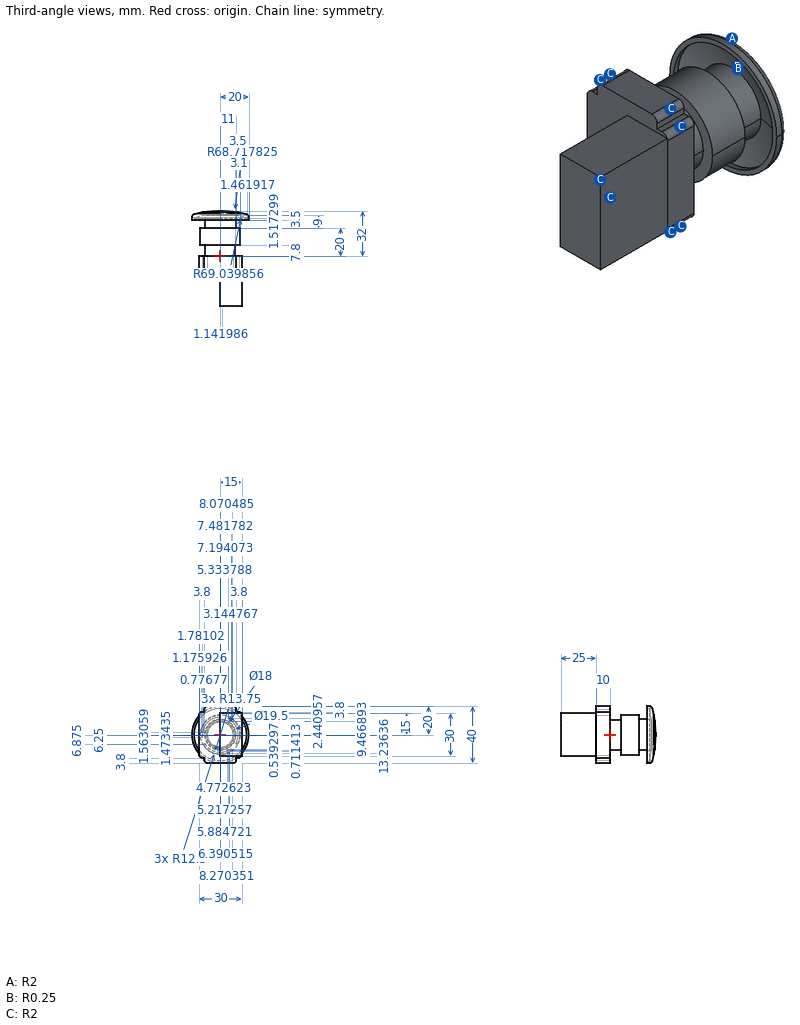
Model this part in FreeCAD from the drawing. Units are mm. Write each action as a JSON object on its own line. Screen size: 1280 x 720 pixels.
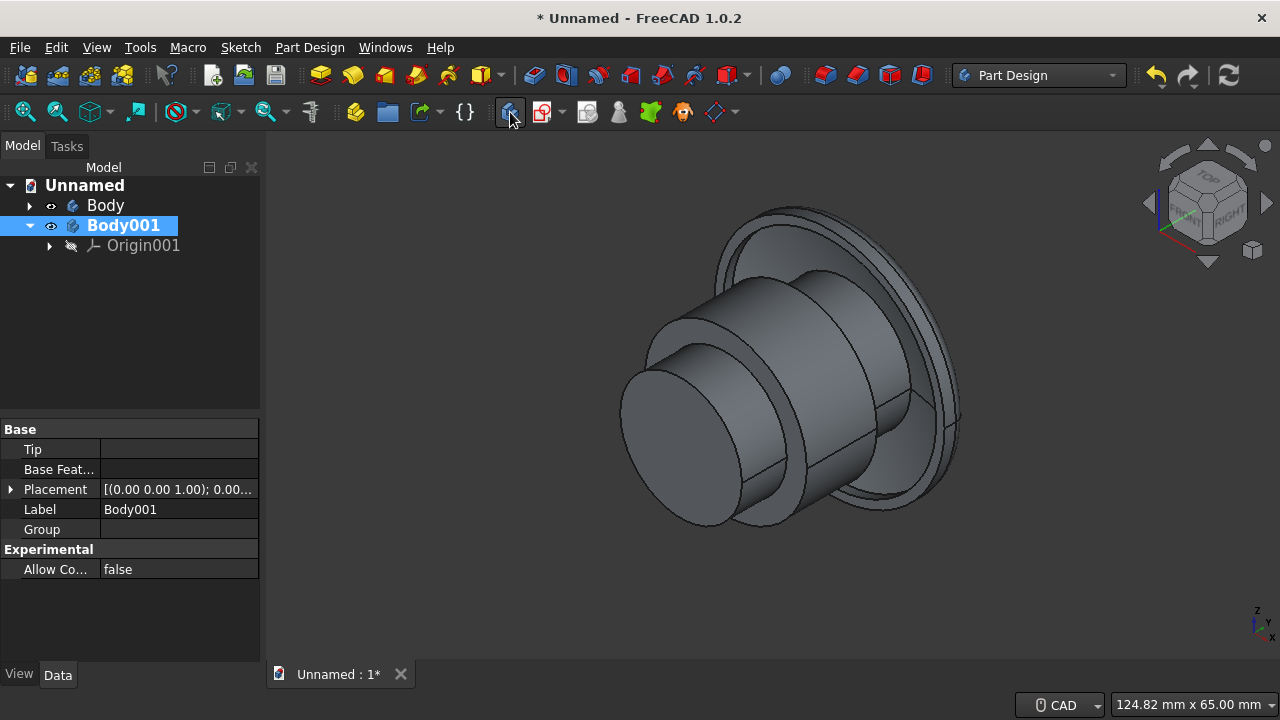
{"action": "left_click", "coordinate": [306, 619]}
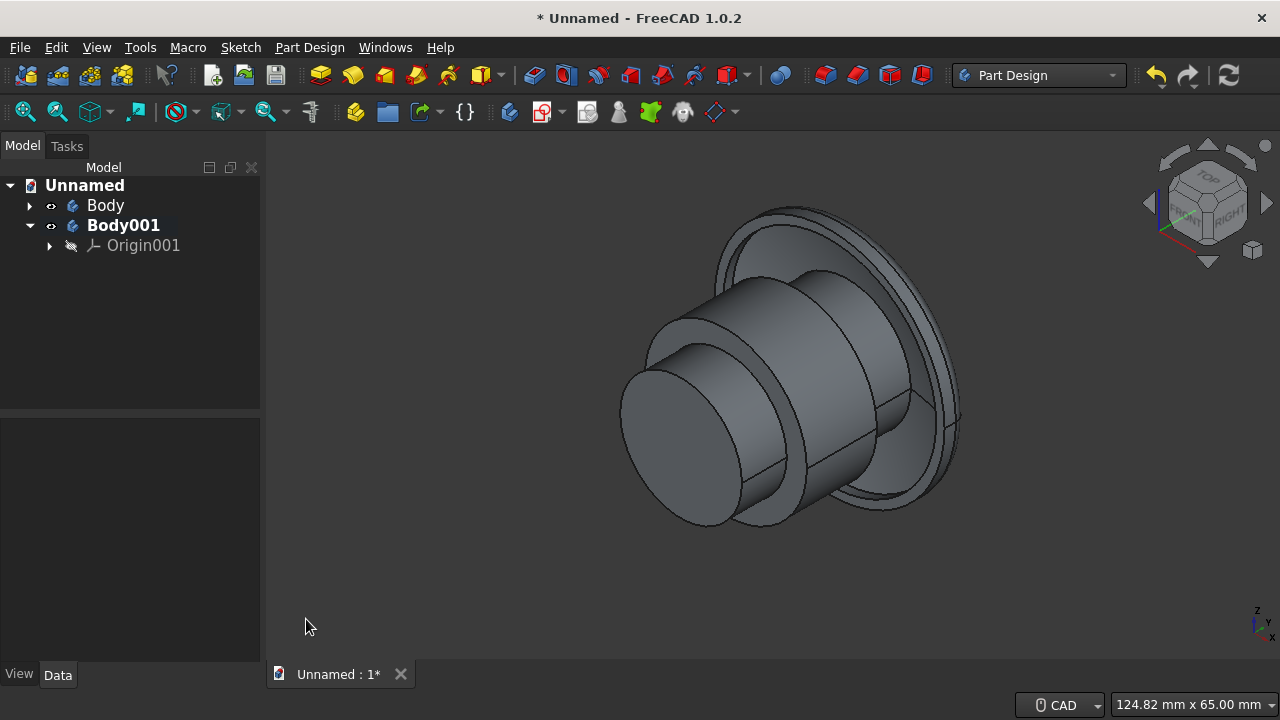
{"action": "left_click", "coordinate": [542, 112]}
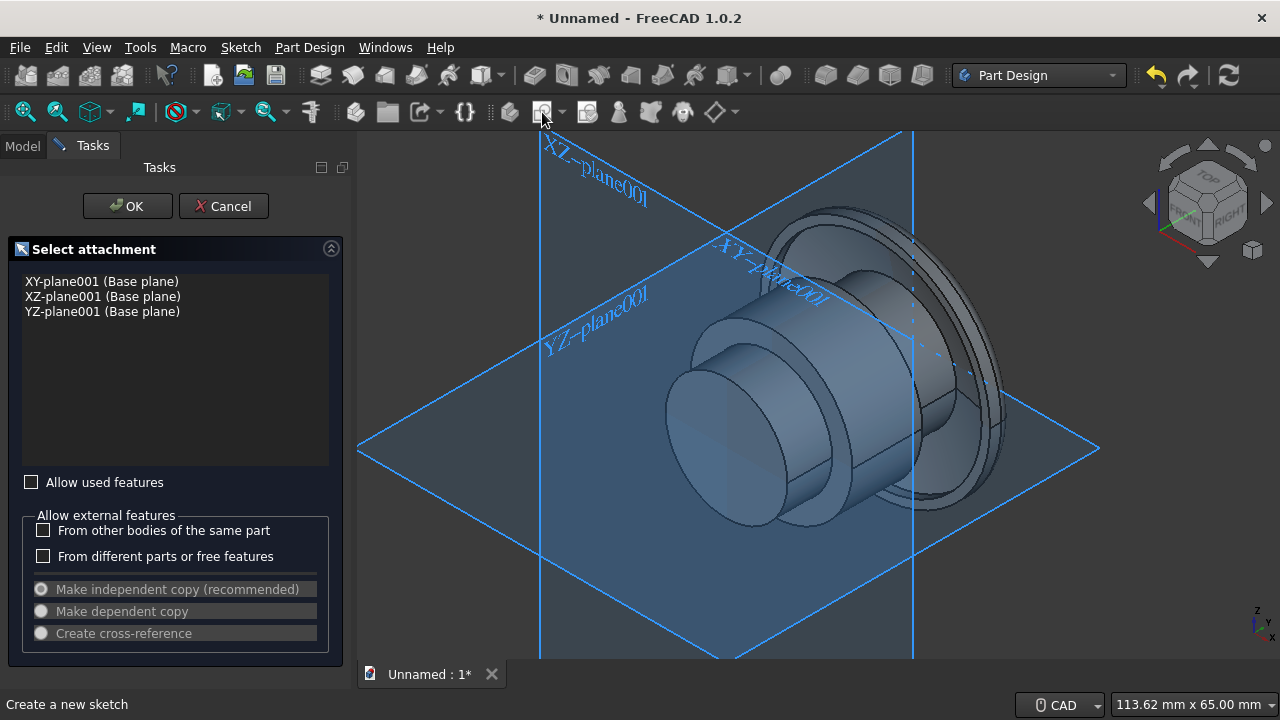
{"action": "left_click", "coordinate": [82, 296]}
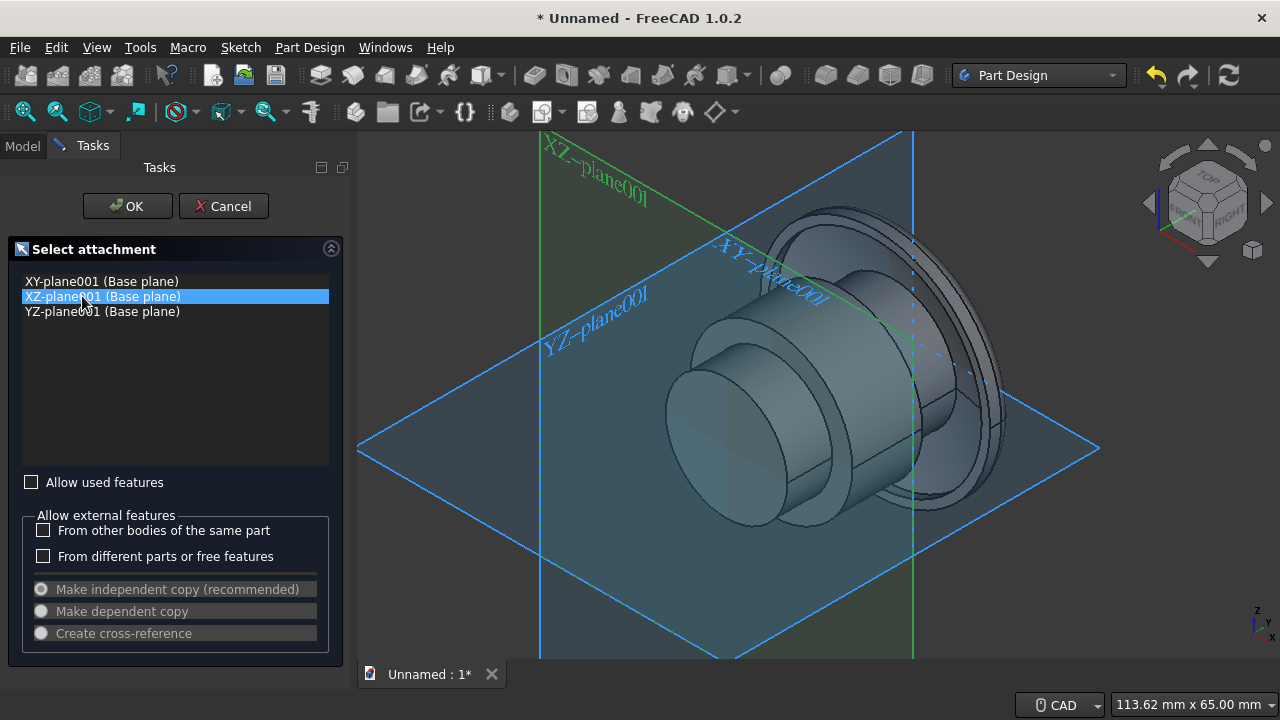
{"action": "left_click", "coordinate": [128, 206]}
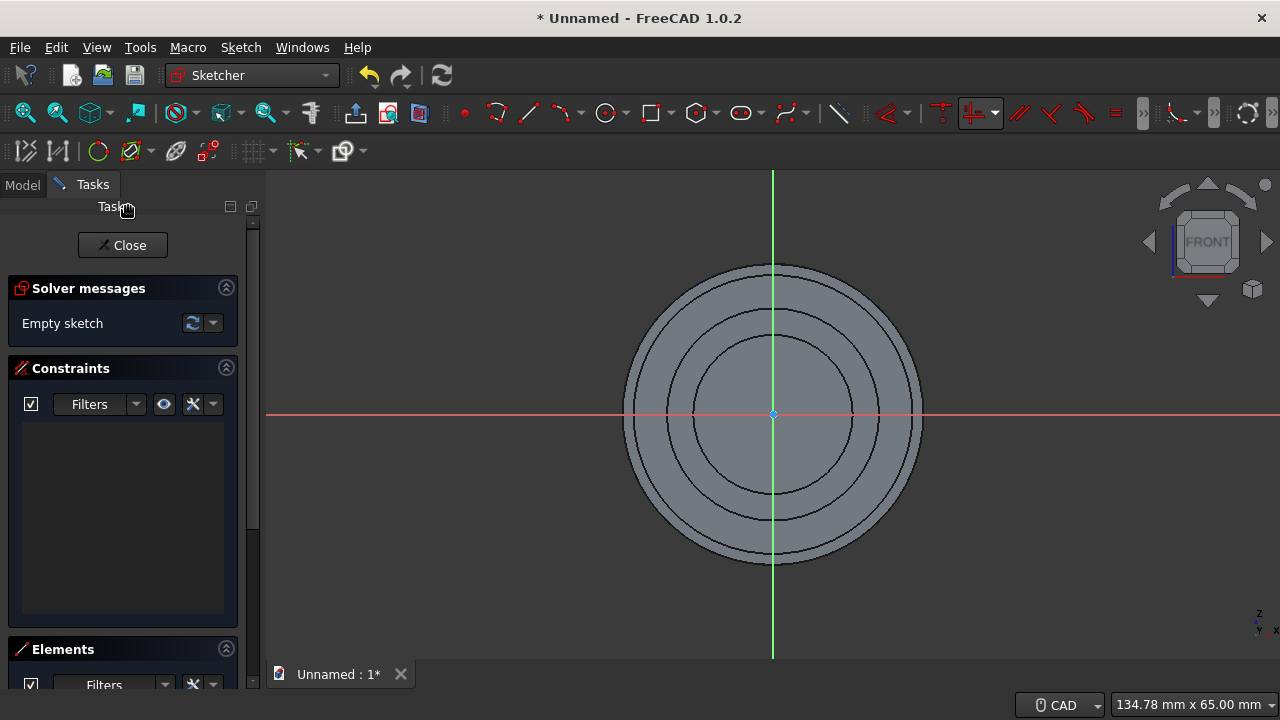
{"action": "left_click", "coordinate": [674, 114]}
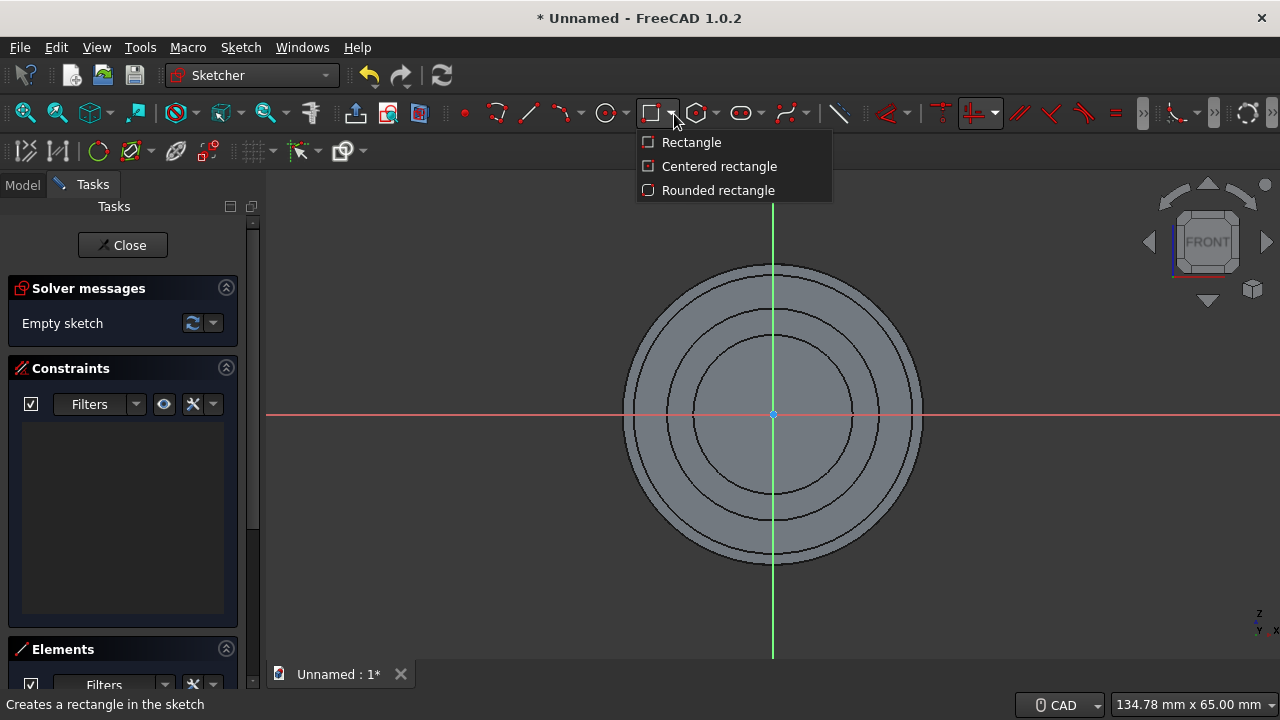
{"action": "left_click", "coordinate": [734, 166]}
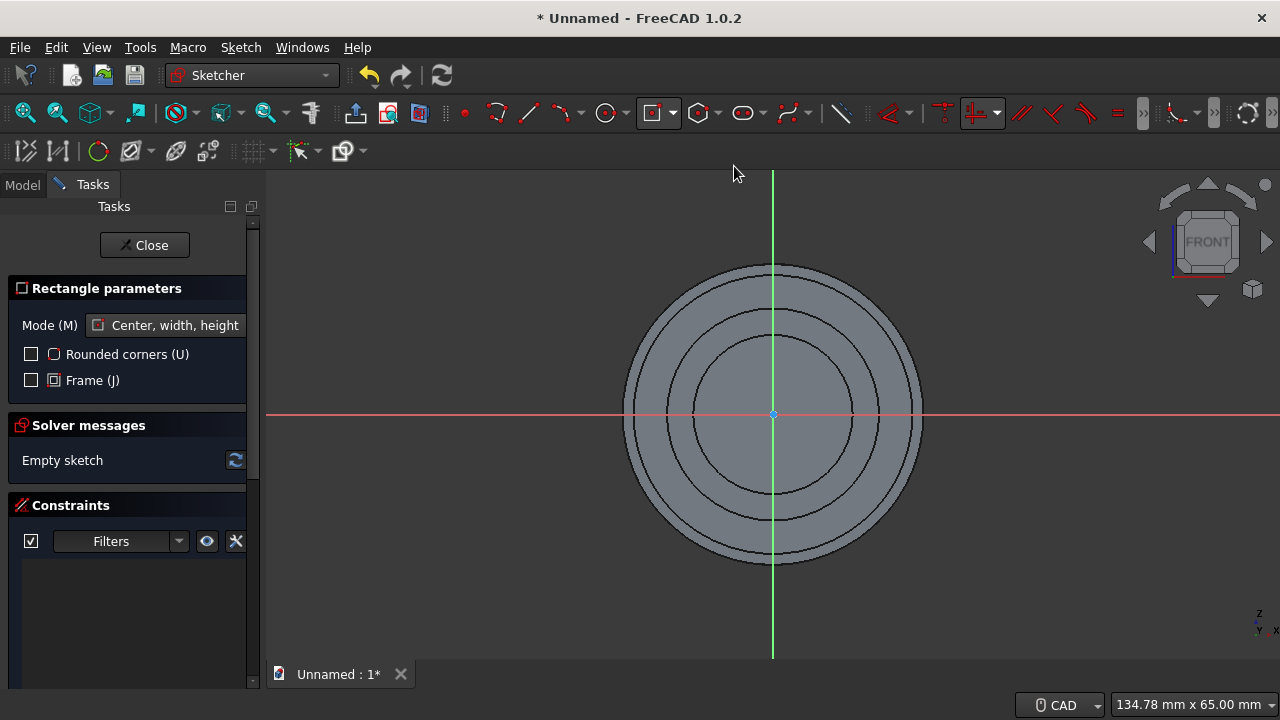
{"action": "left_click", "coordinate": [773, 414]}
{"action": "mouse_move", "coordinate": [886, 264]}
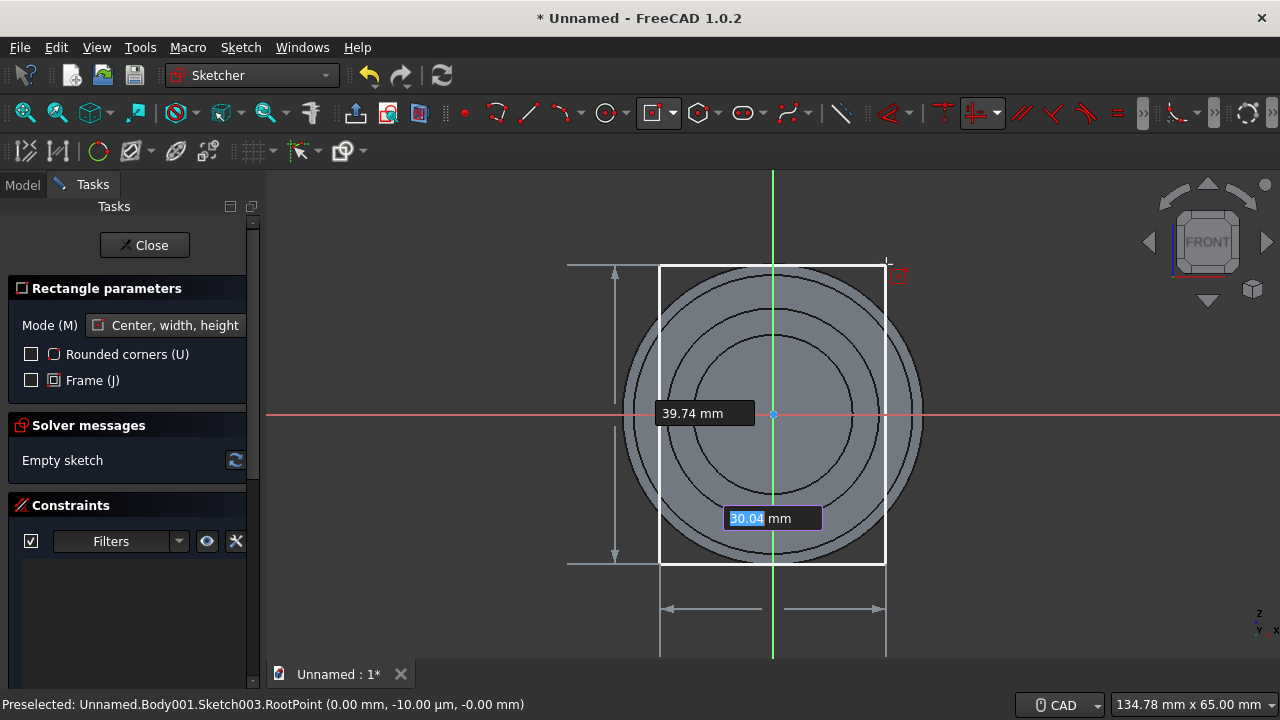
{"action": "type", "text": "30"}
{"action": "key", "text": "Tab"}
{"action": "type", "text": "40"}
{"action": "key", "text": "Return"}
{"action": "key", "text": "Escape"}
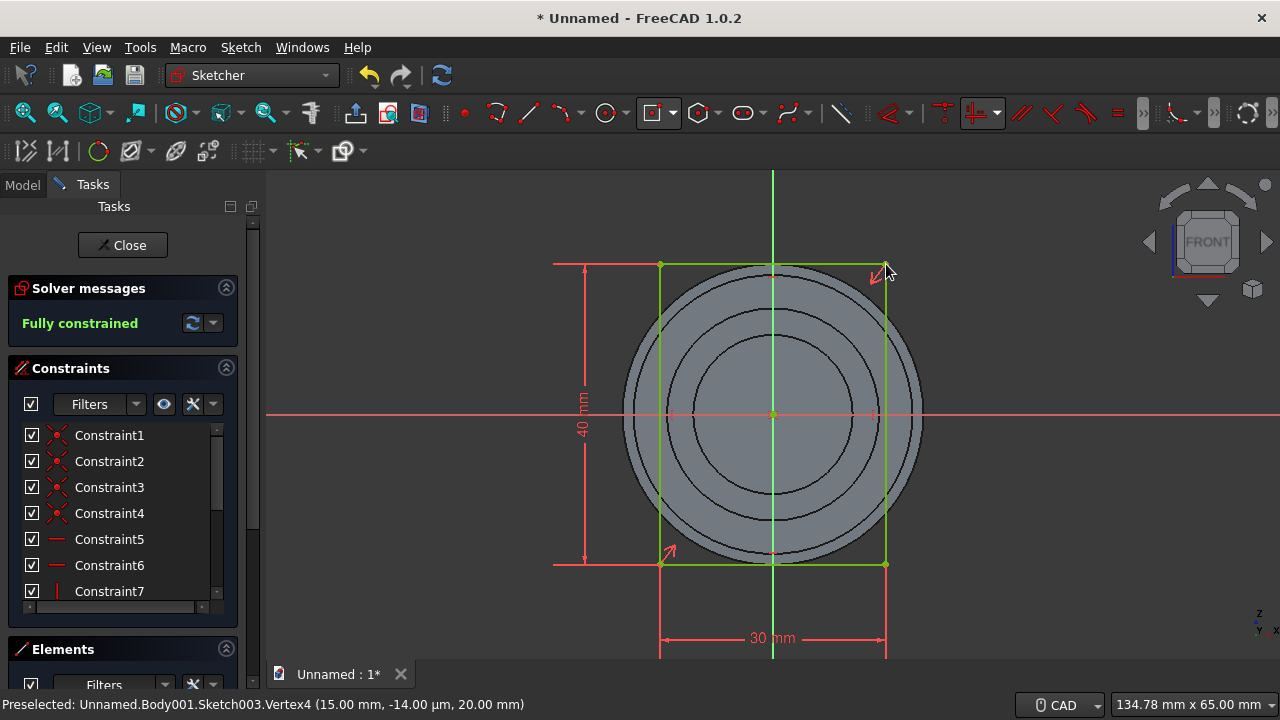
{"action": "left_click", "coordinate": [123, 245]}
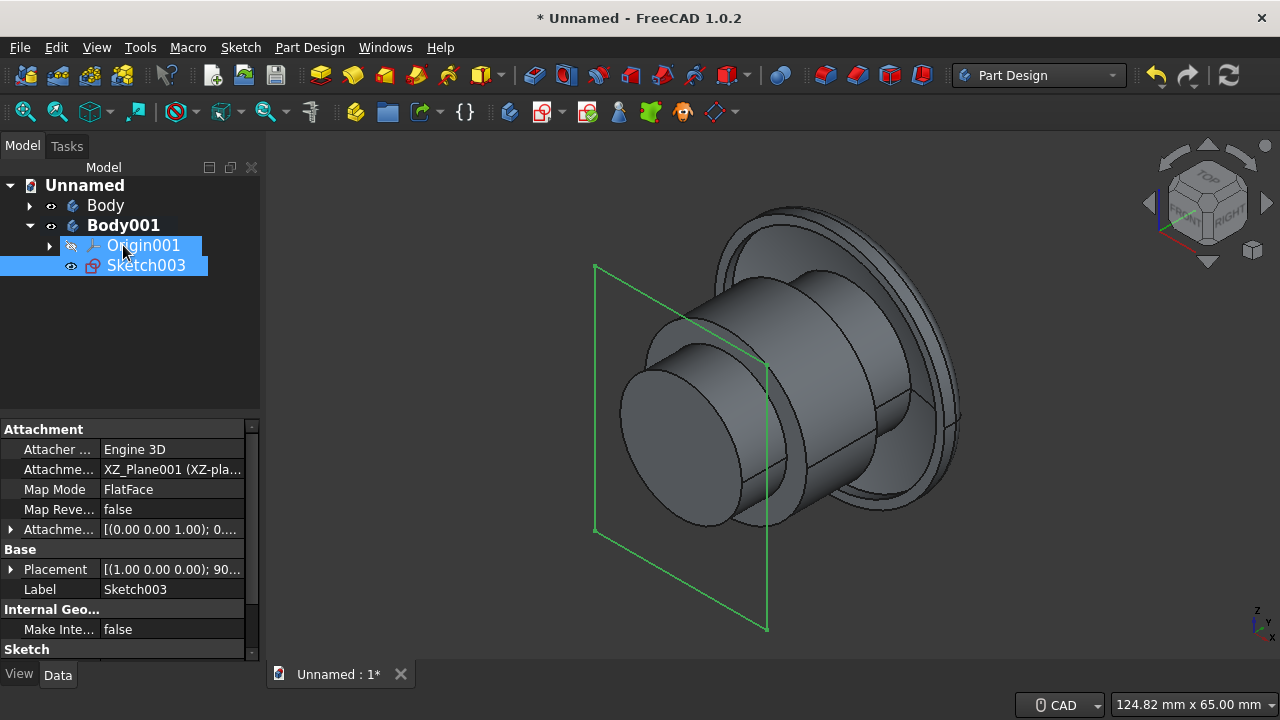
{"action": "left_click", "coordinate": [322, 76]}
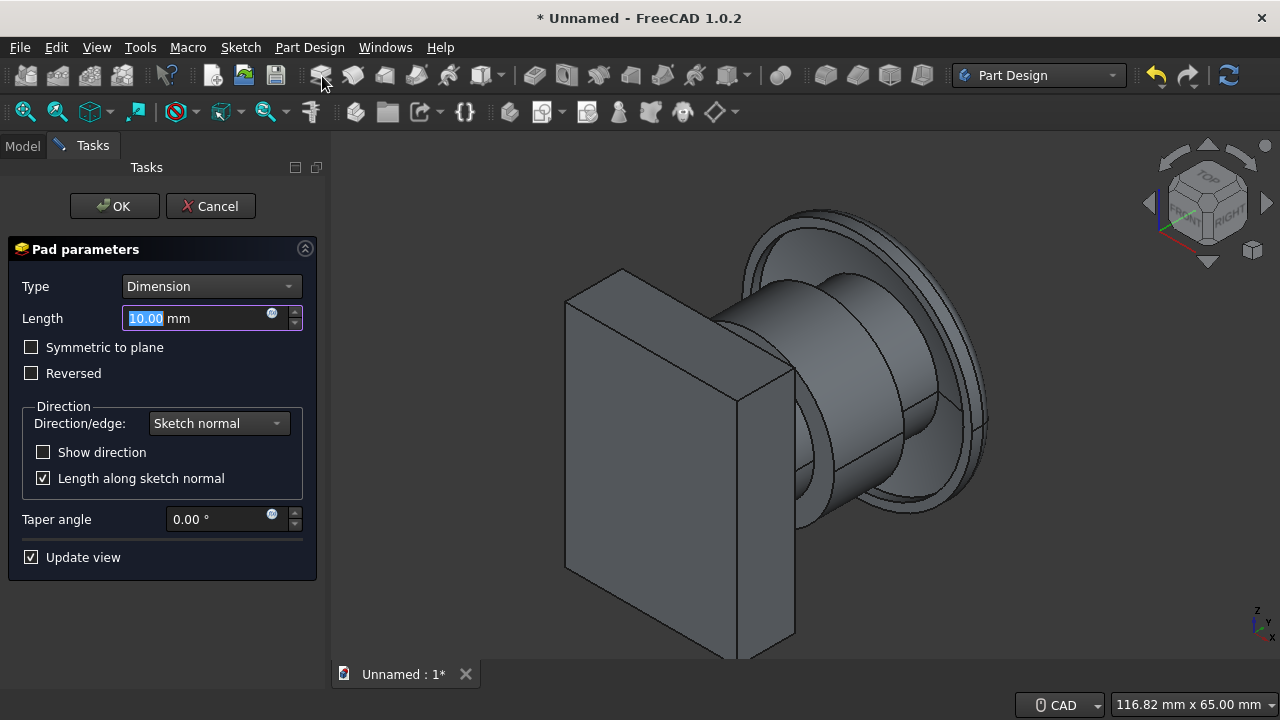
{"action": "type", "text": "10"}
{"action": "key", "text": "Tab"}